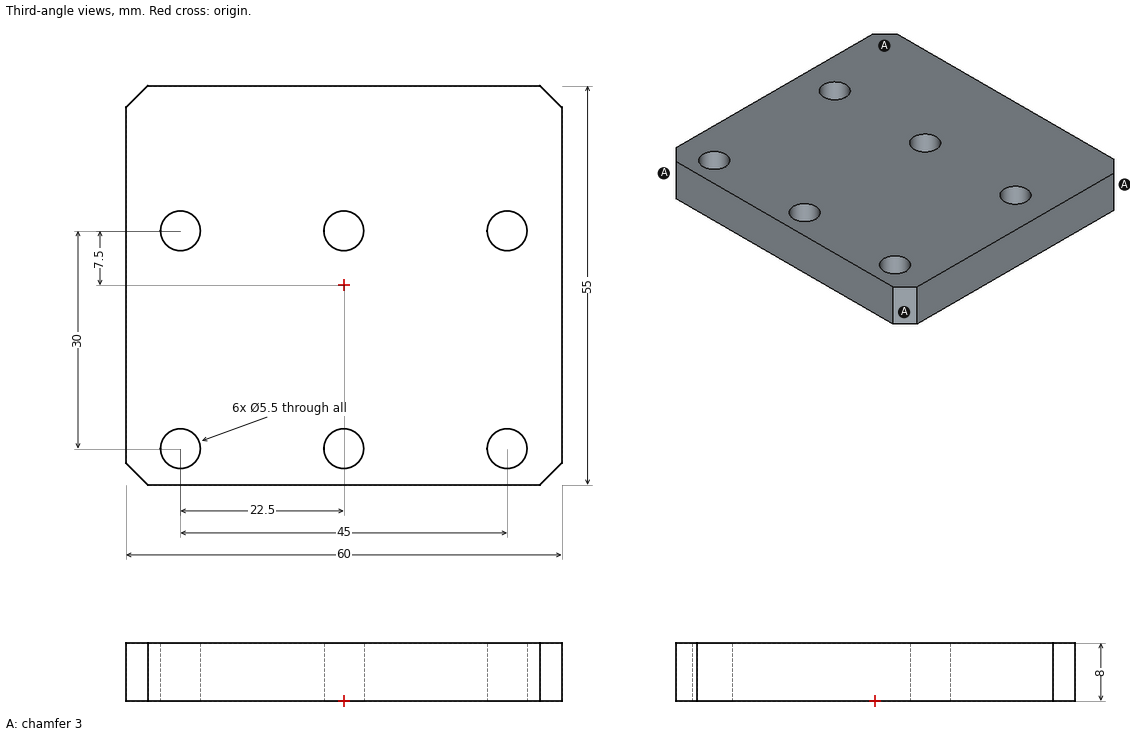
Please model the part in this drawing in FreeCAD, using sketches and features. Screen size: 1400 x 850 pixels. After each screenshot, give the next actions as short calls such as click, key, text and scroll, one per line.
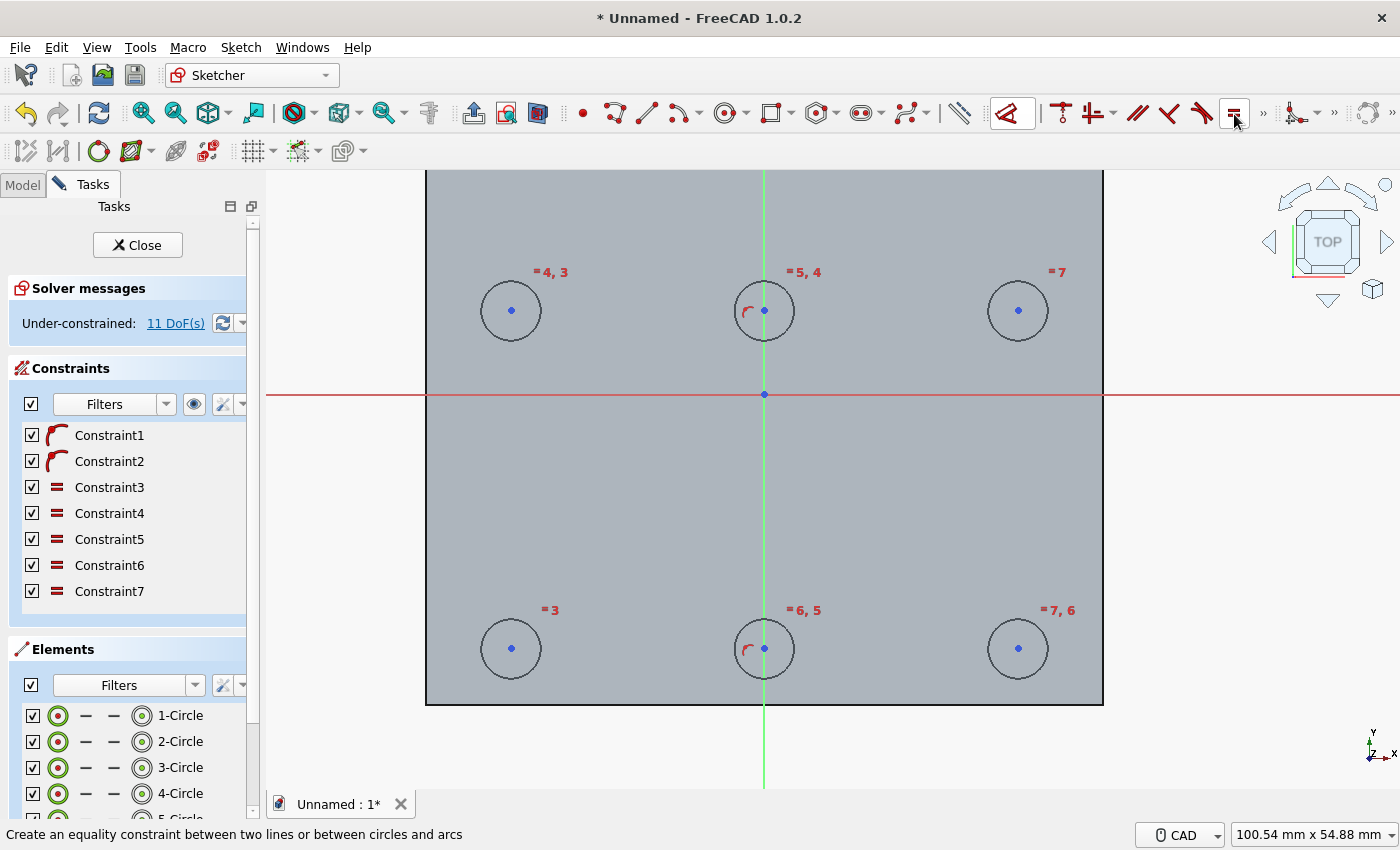
click(511, 649)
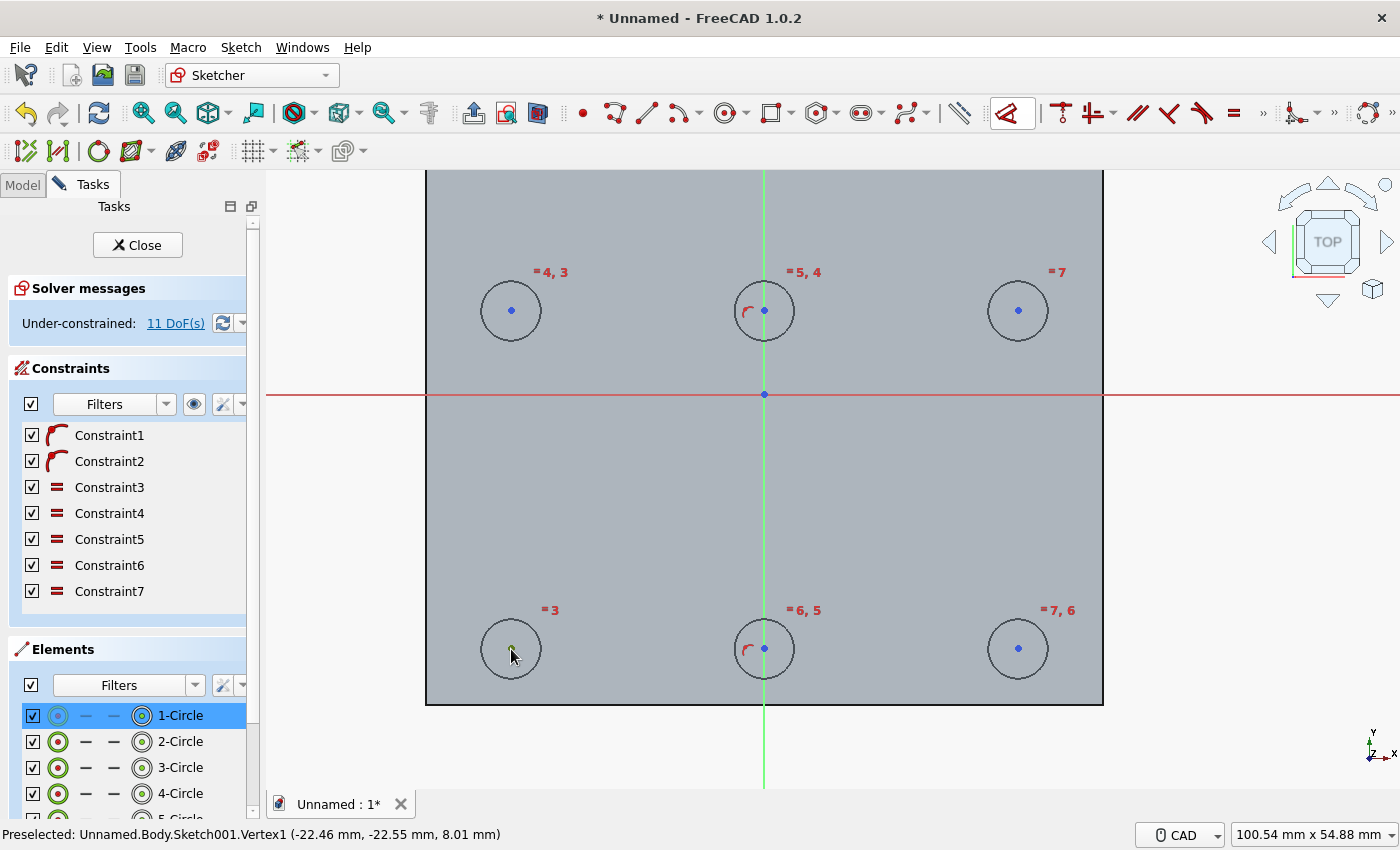
click(511, 311)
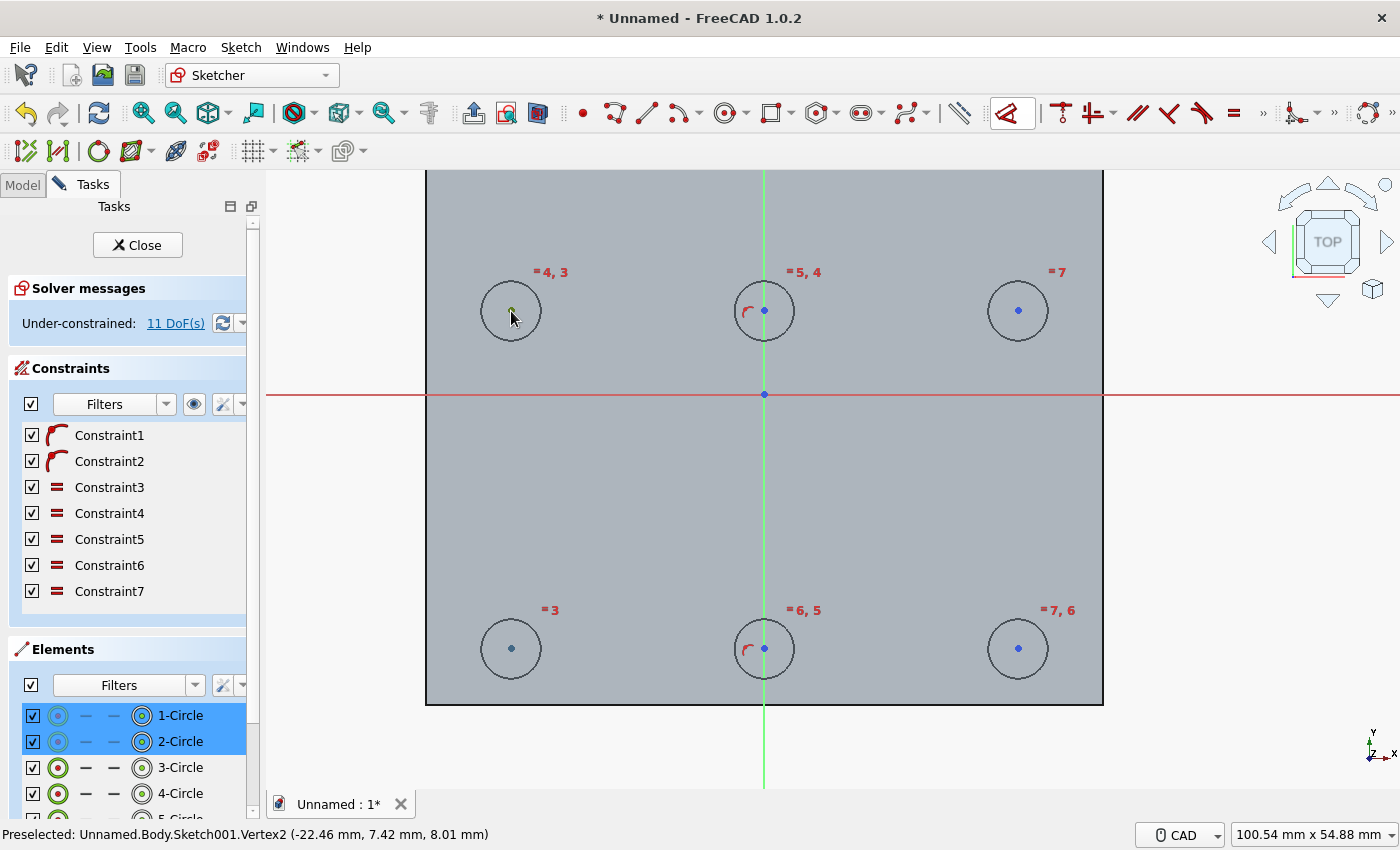
click(1116, 114)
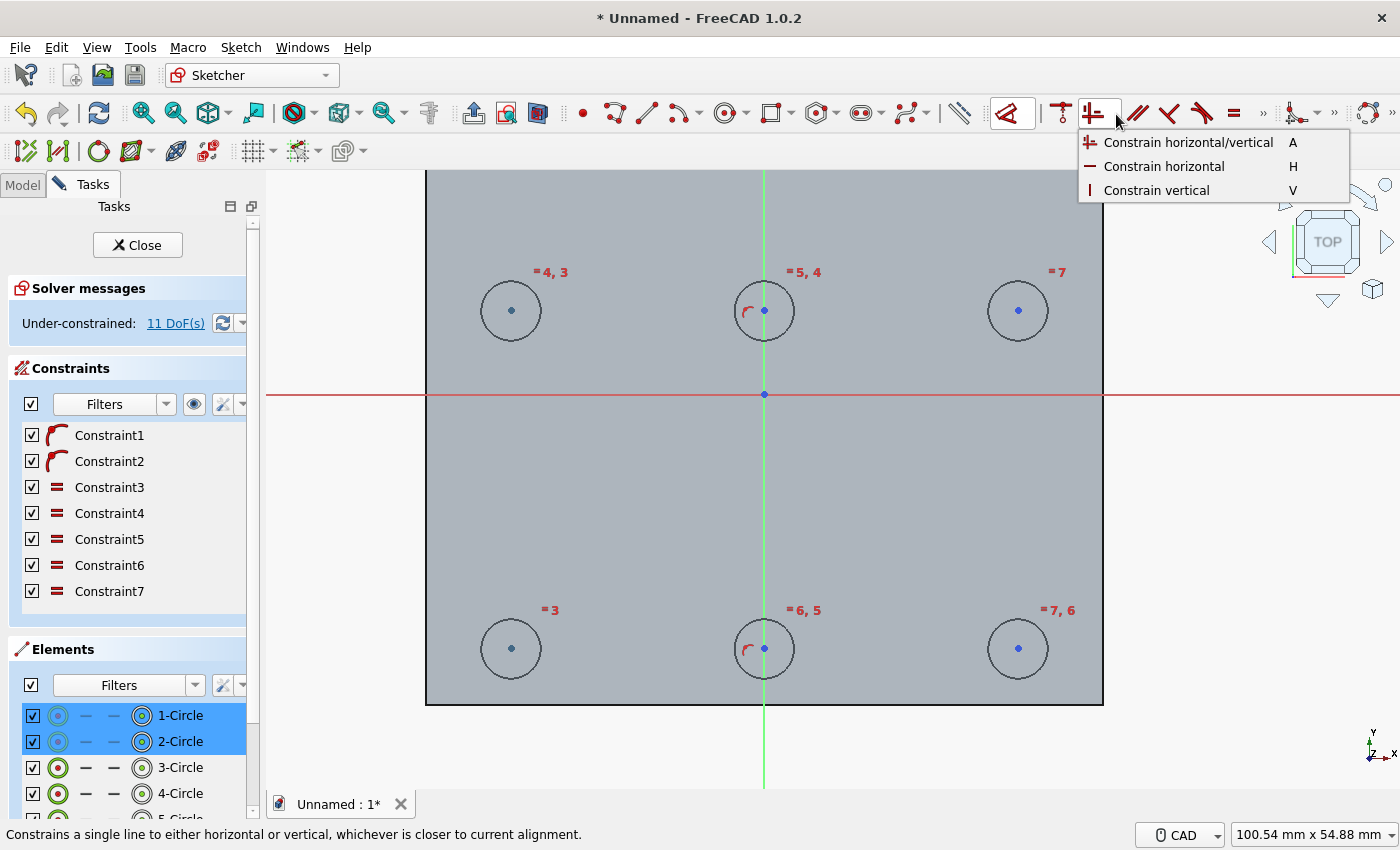
click(1214, 190)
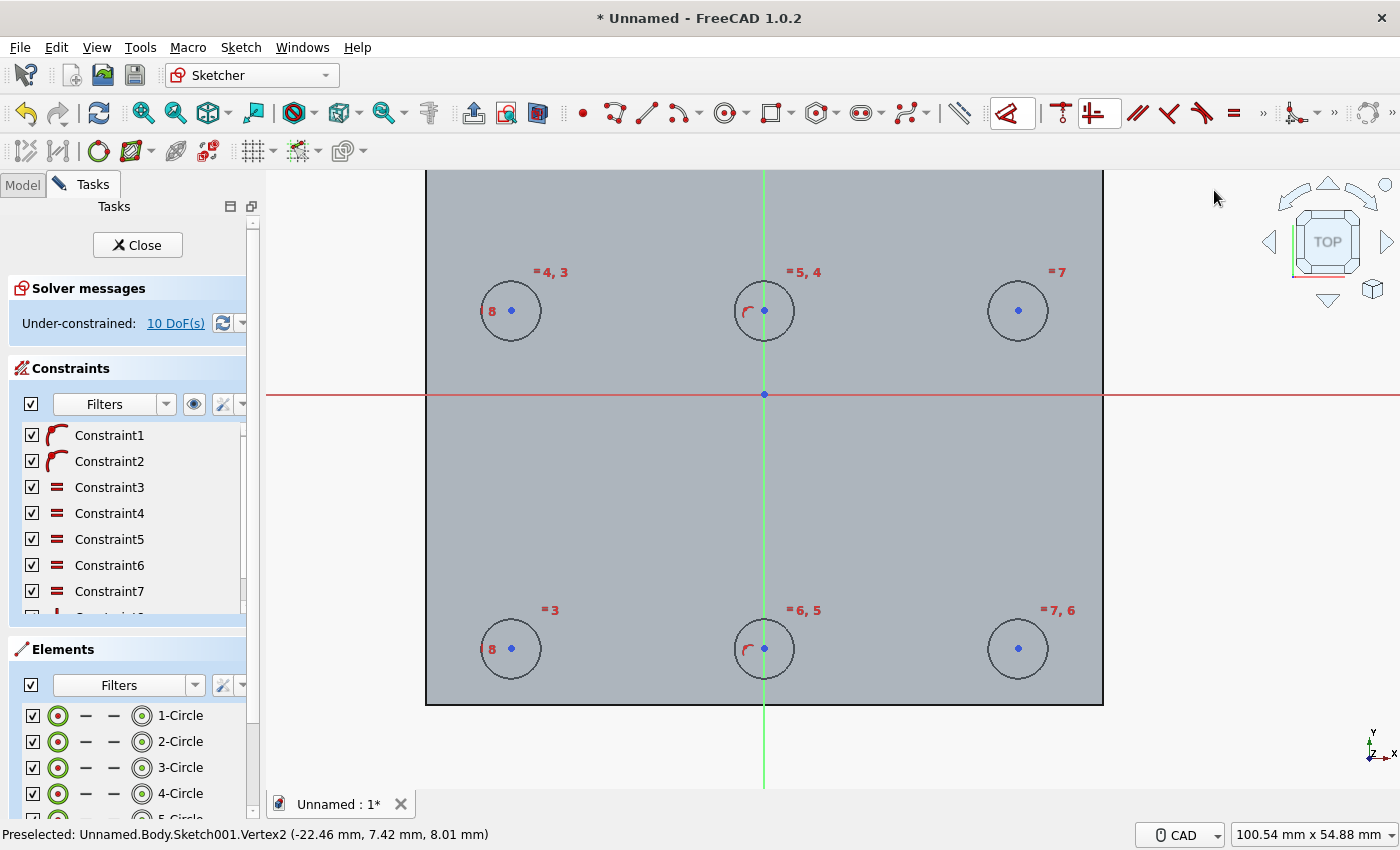
click(511, 311)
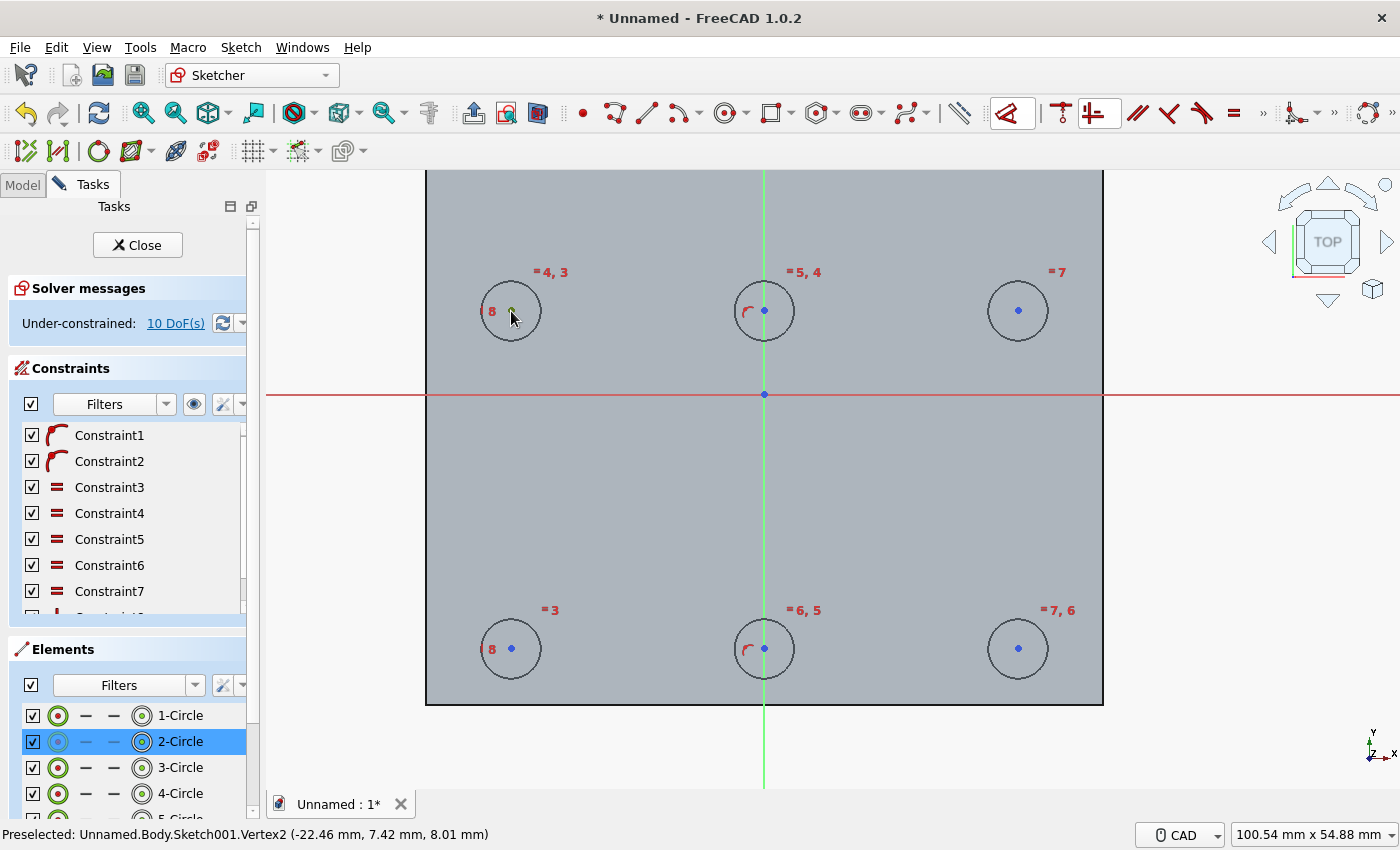
click(764, 311)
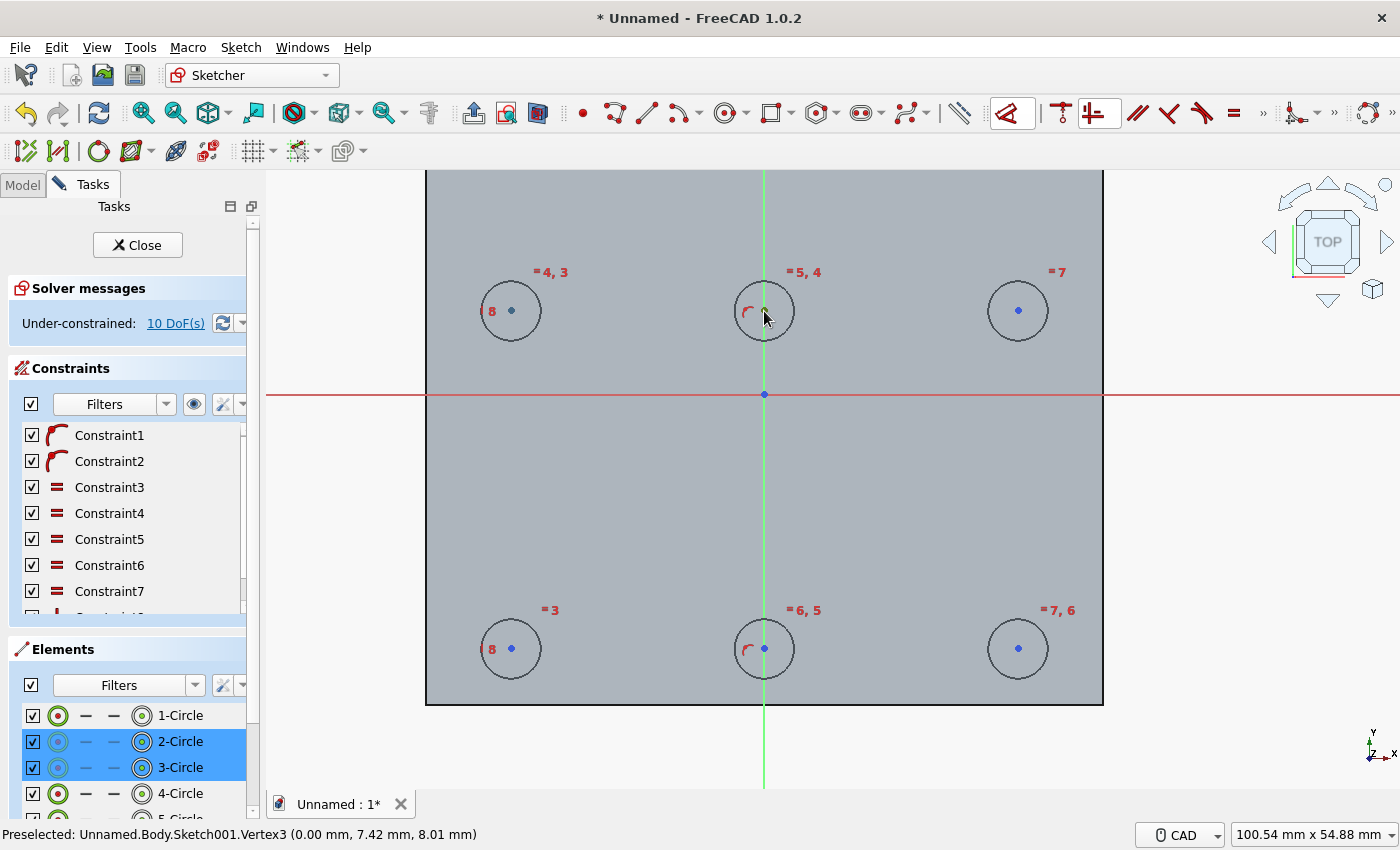
key(h)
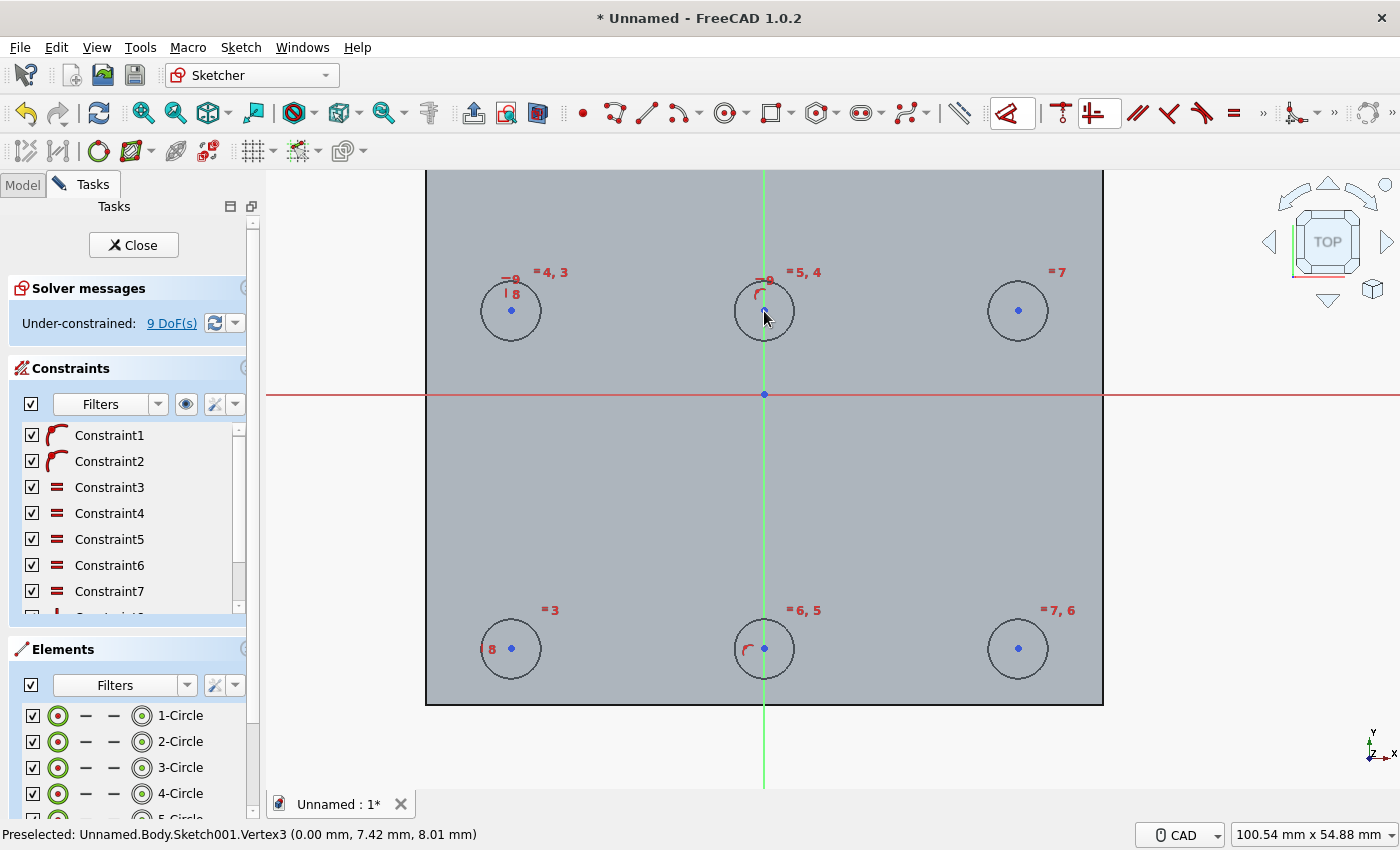
click(511, 649)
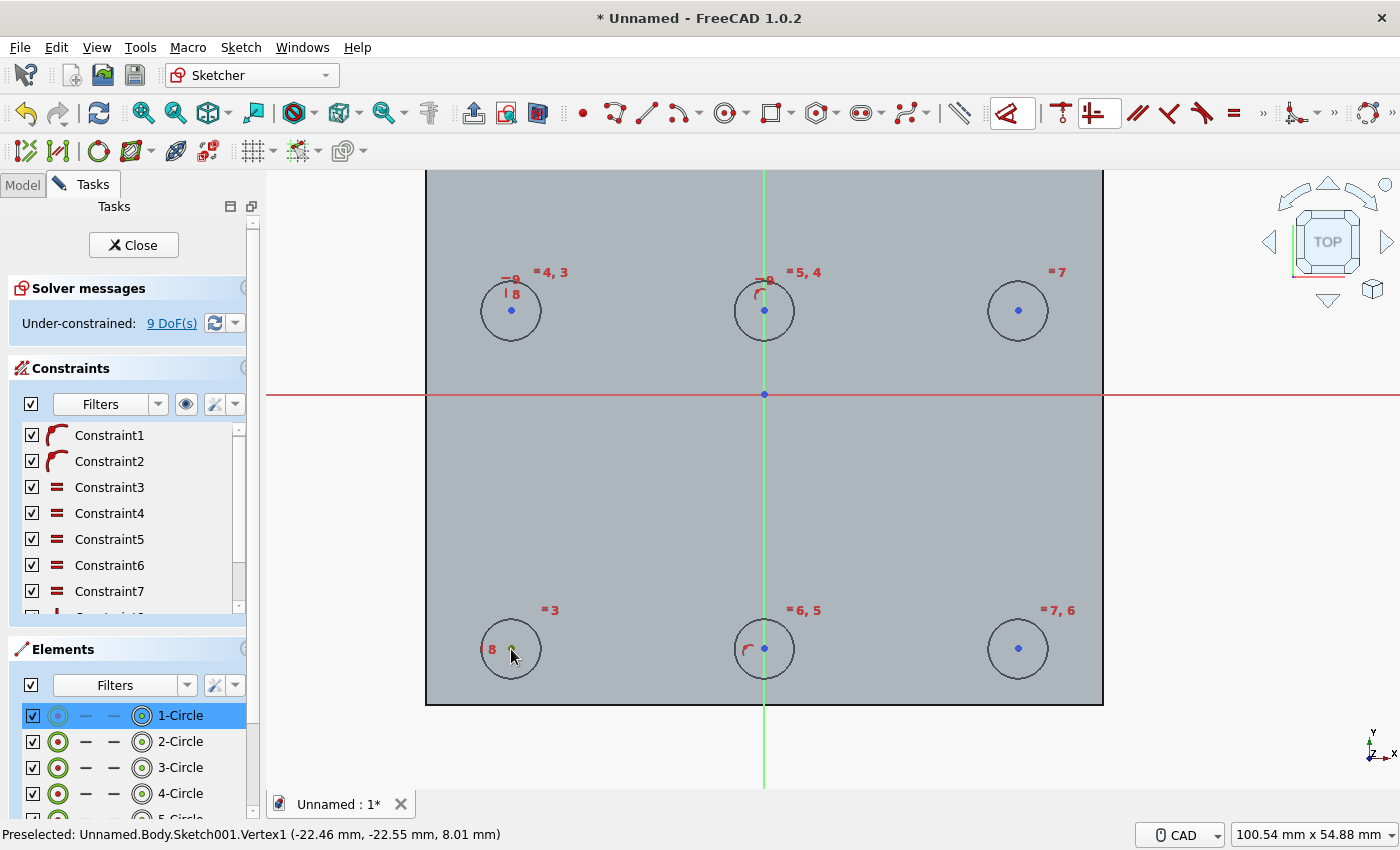
click(764, 649)